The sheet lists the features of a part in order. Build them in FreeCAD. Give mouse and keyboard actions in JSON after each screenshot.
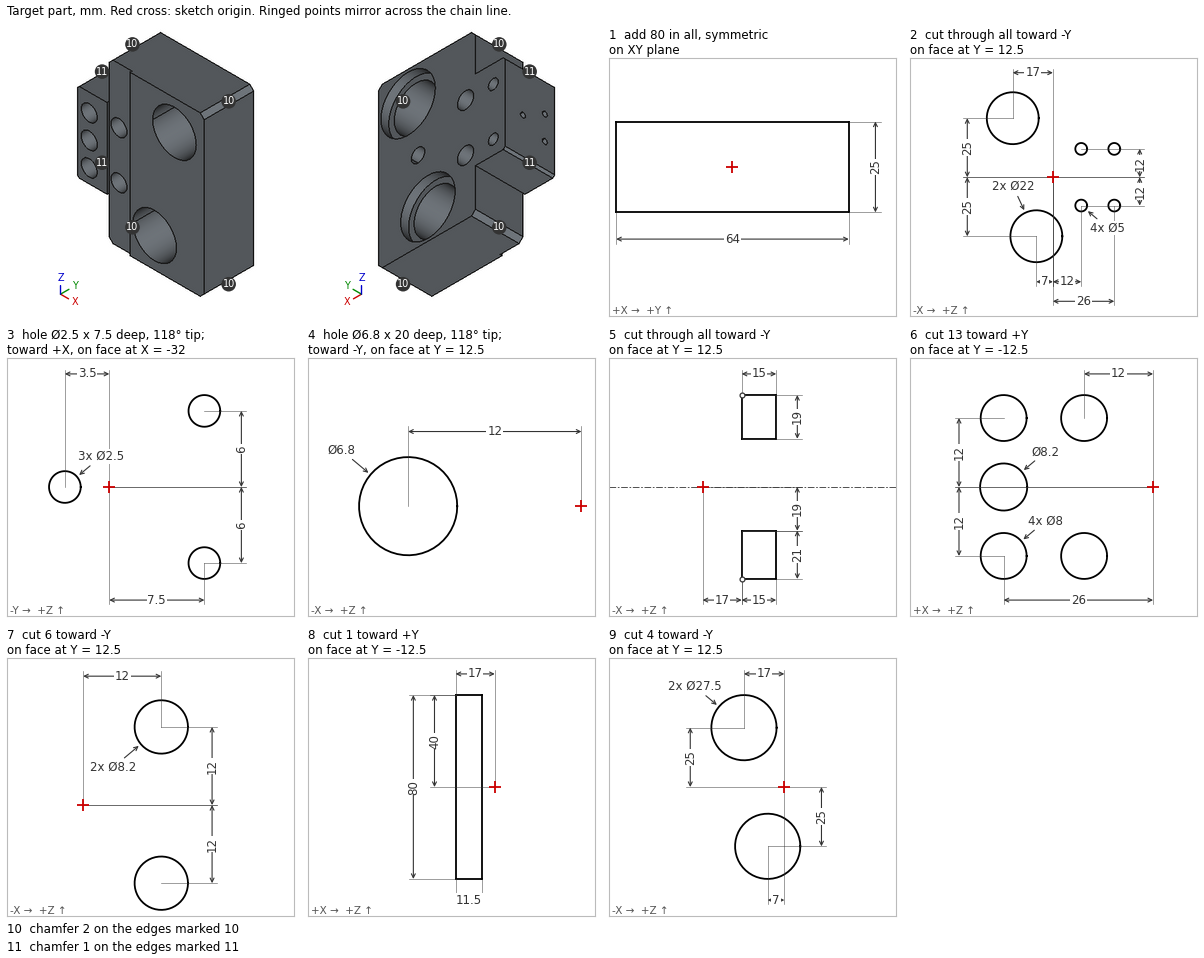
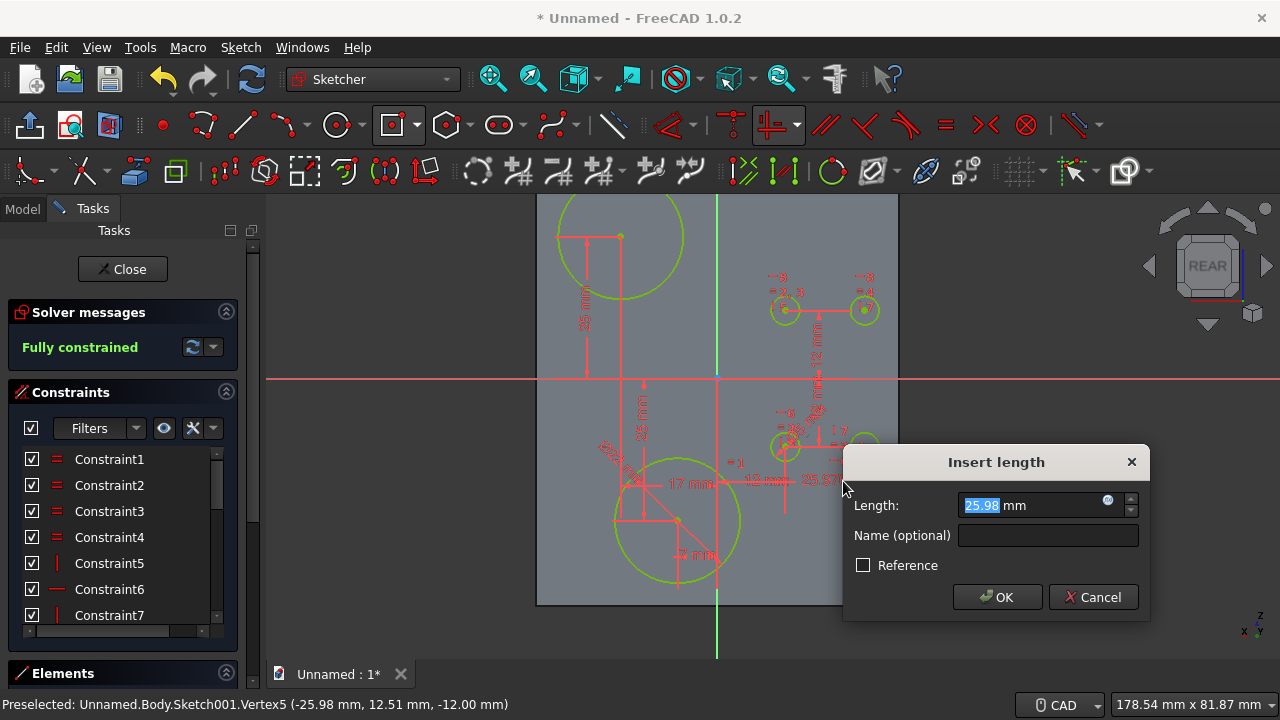
{"action": "type", "text": "26"}
{"action": "key", "text": "Return"}
{"action": "key", "text": "Escape"}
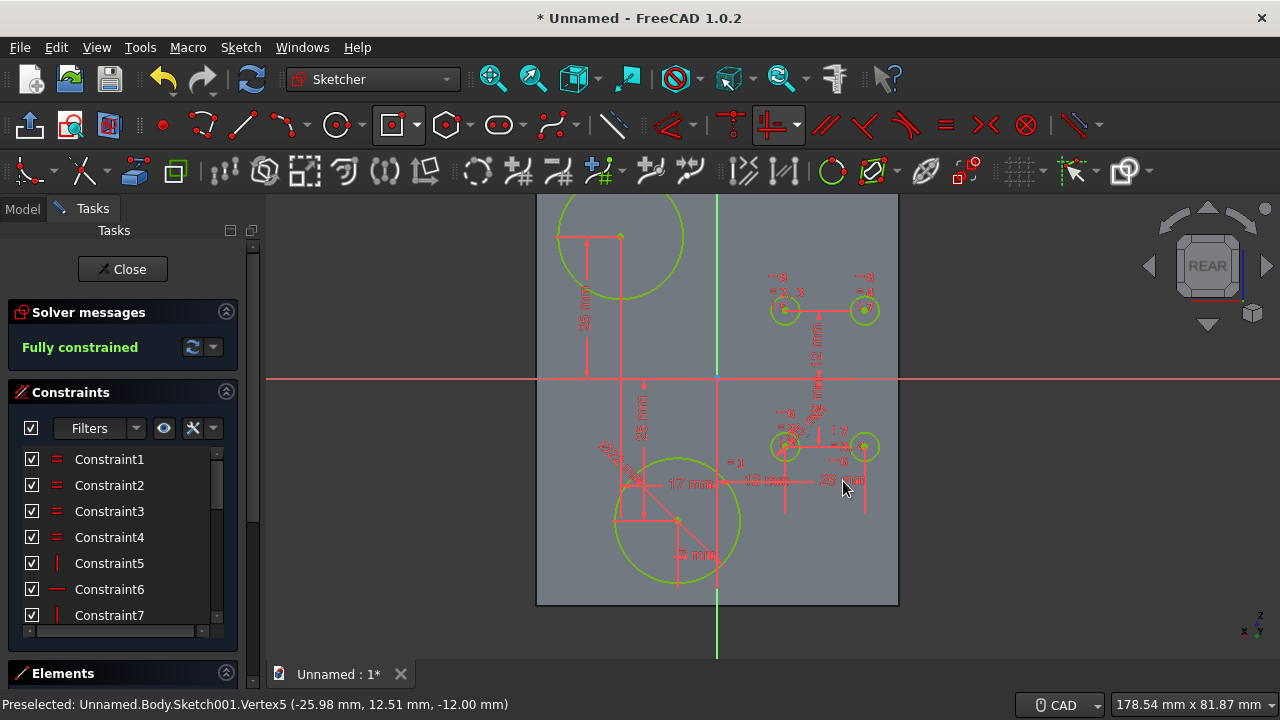
{"action": "left_click", "coordinate": [123, 269]}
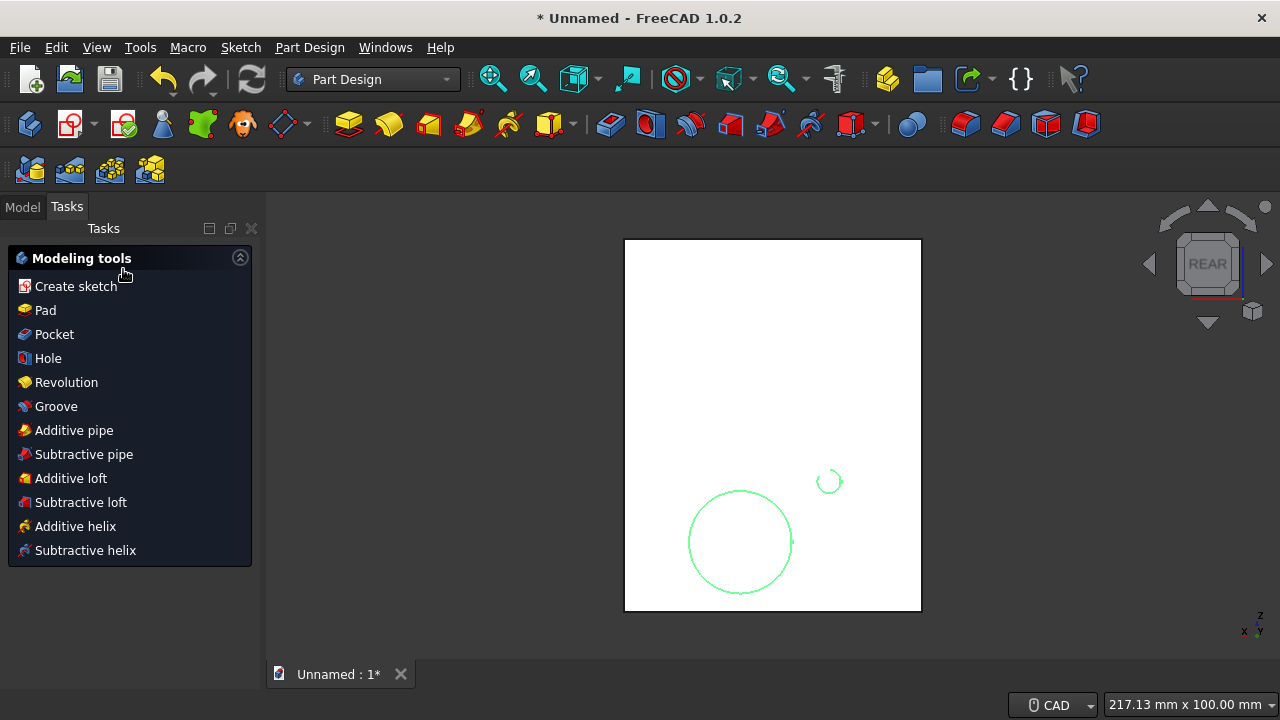
{"action": "left_click", "coordinate": [612, 124]}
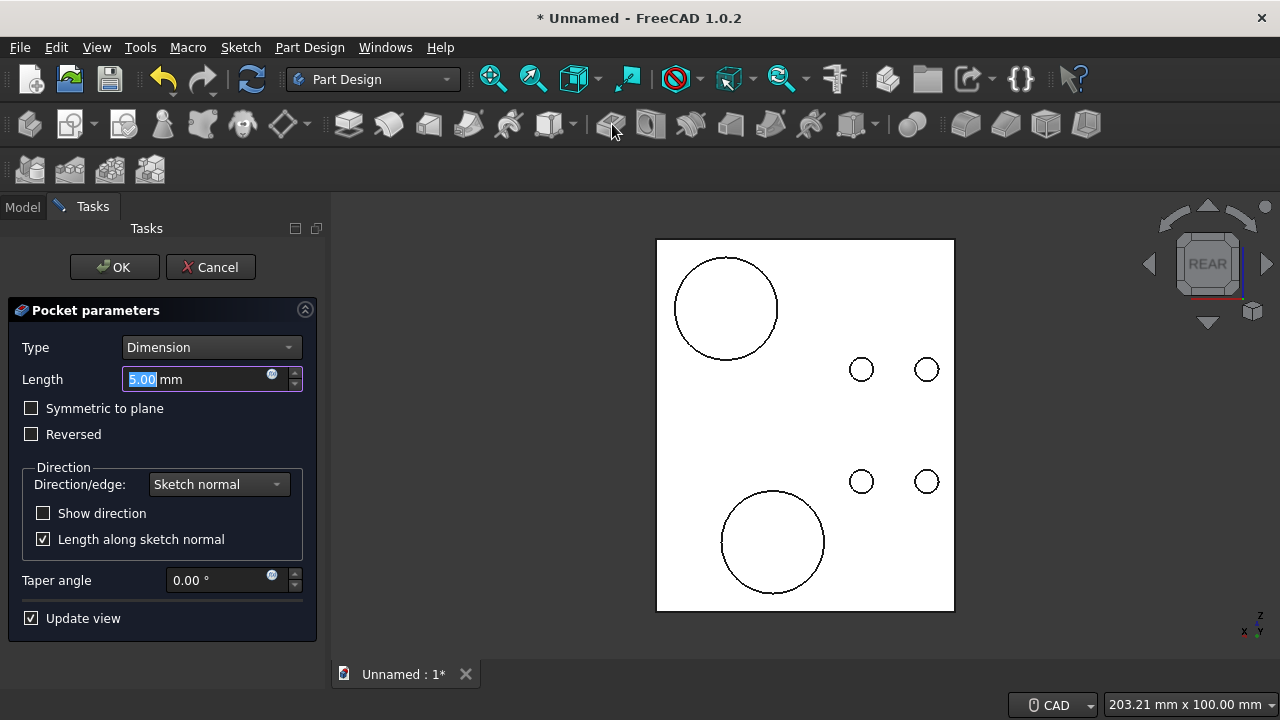
{"action": "left_click", "coordinate": [212, 348]}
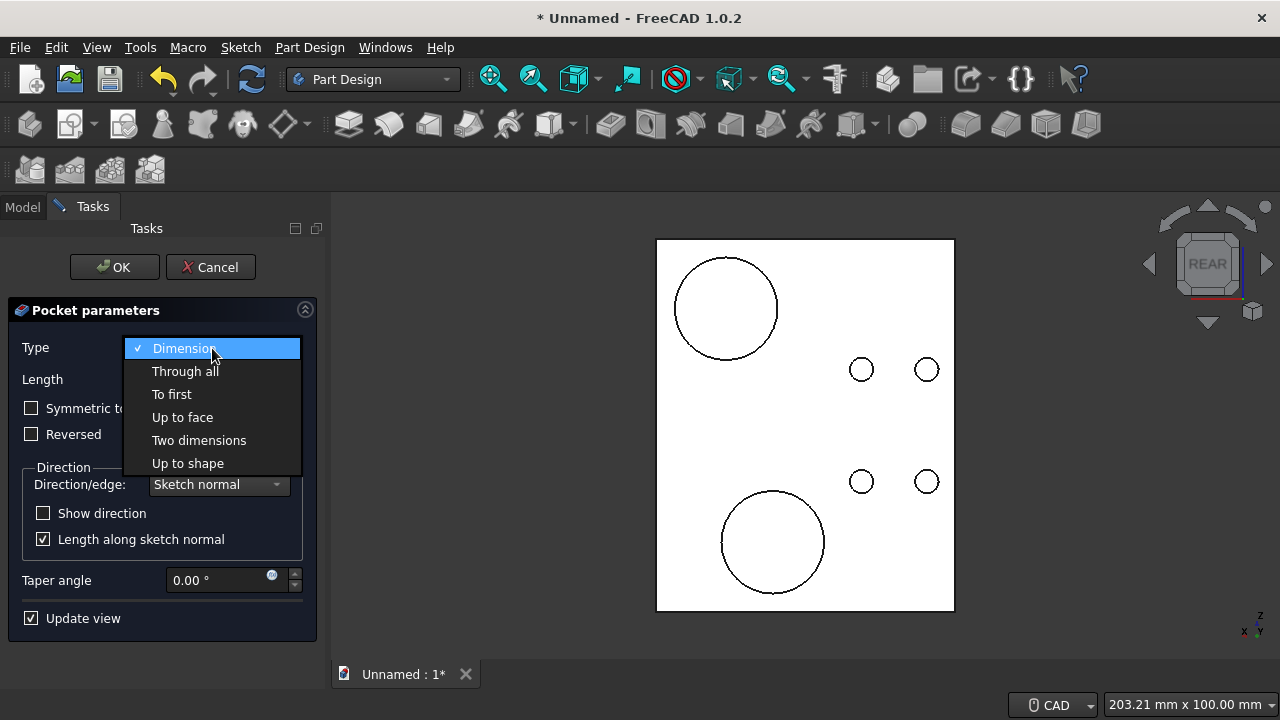
{"action": "left_click", "coordinate": [212, 372]}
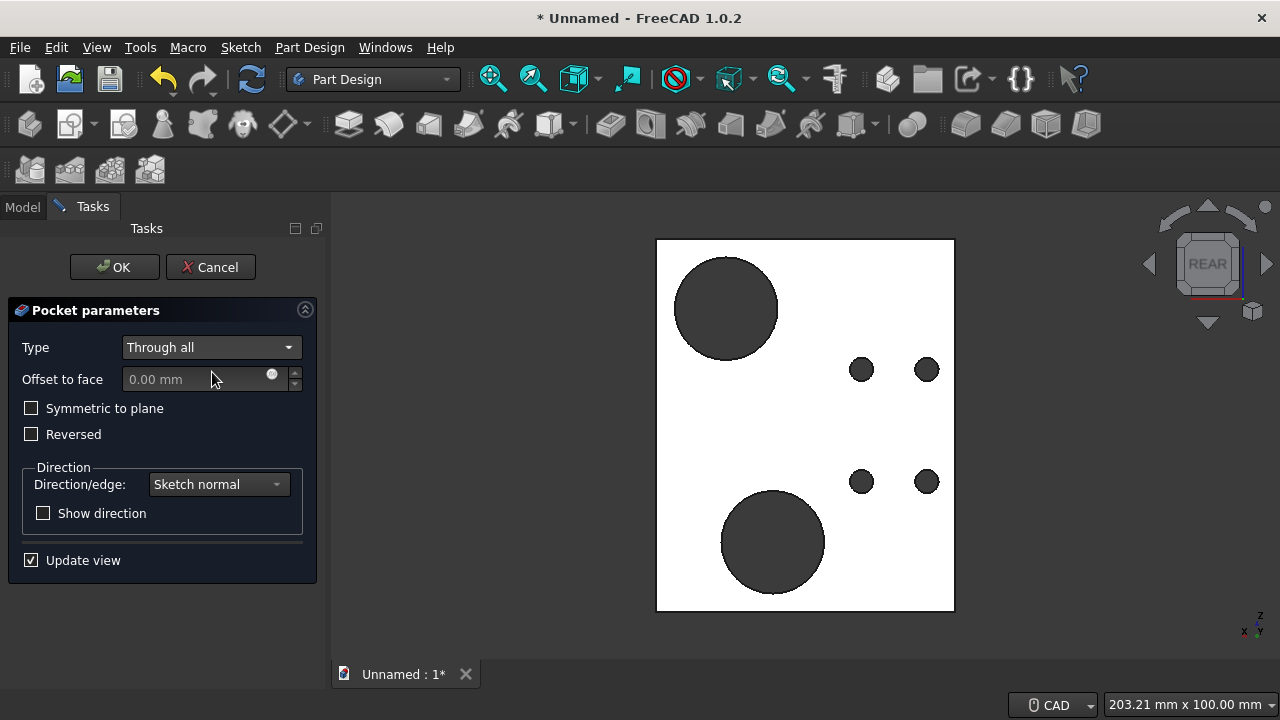
{"action": "left_click", "coordinate": [115, 267]}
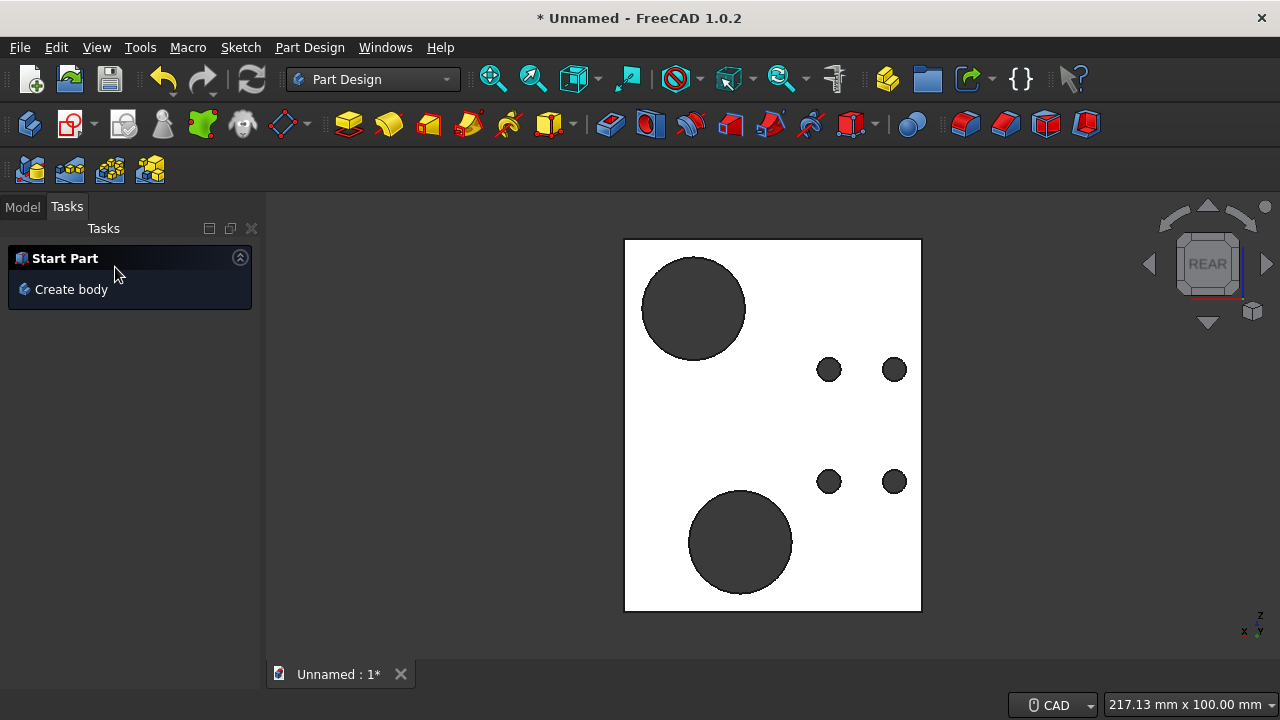
{"action": "key", "text": "6"}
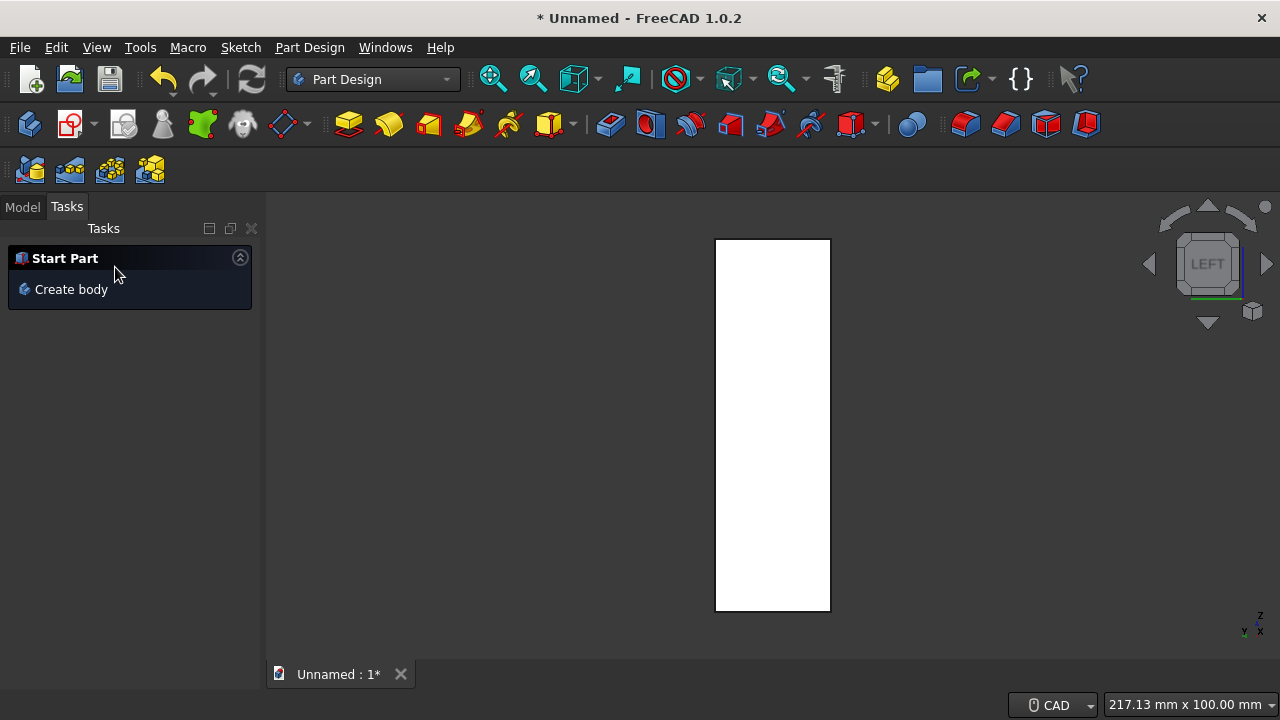
{"action": "left_click", "coordinate": [773, 318]}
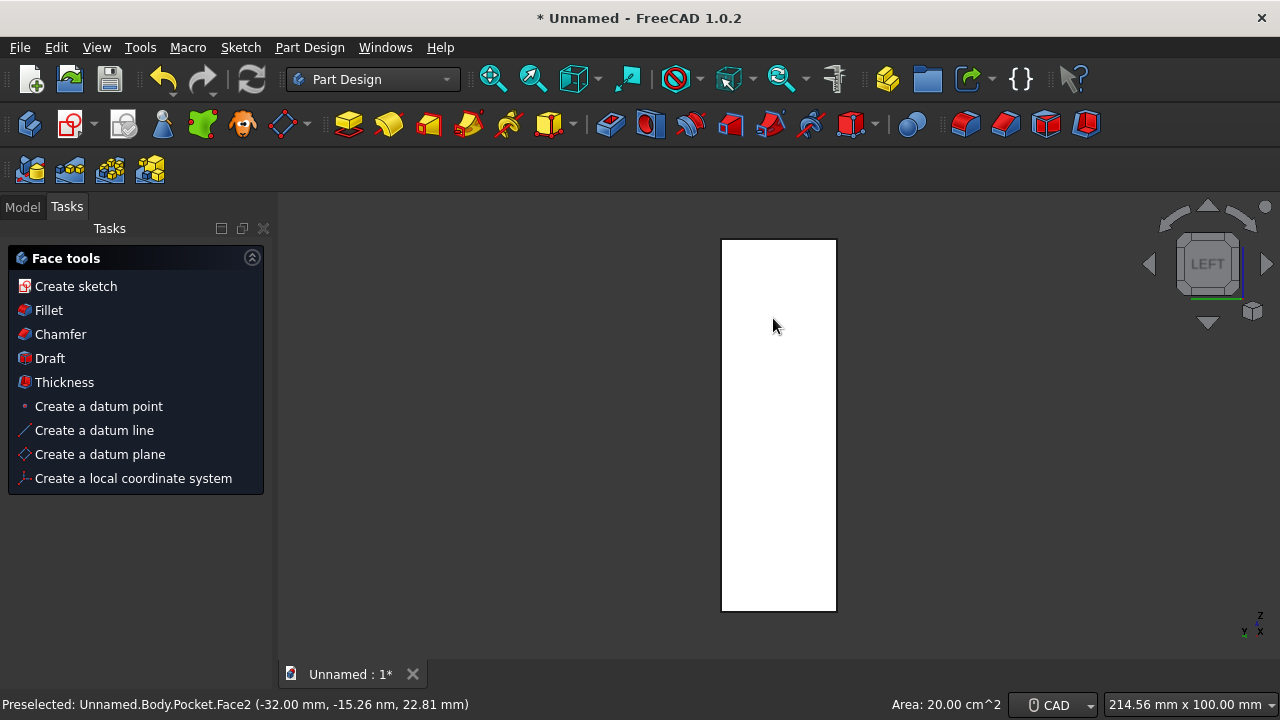
{"action": "left_click", "coordinate": [70, 124]}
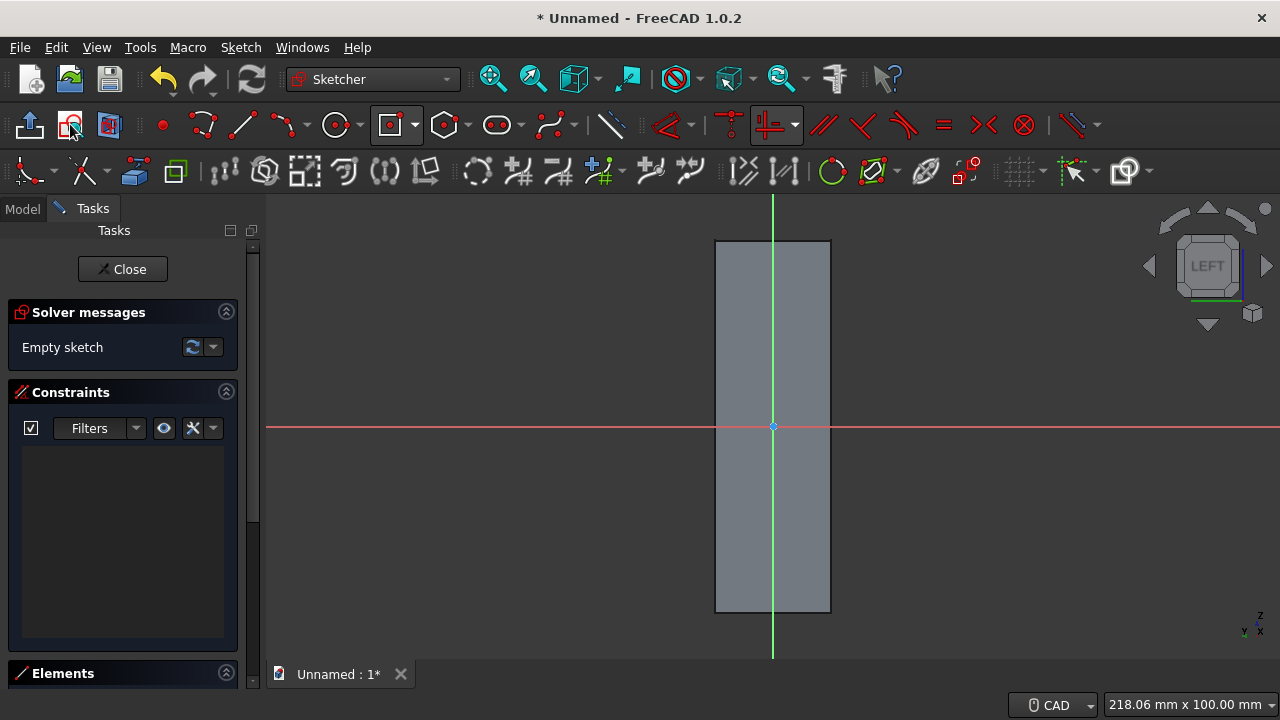
{"action": "scroll", "coordinate": [808, 427], "scroll_direction": "up", "scroll_amount": 7}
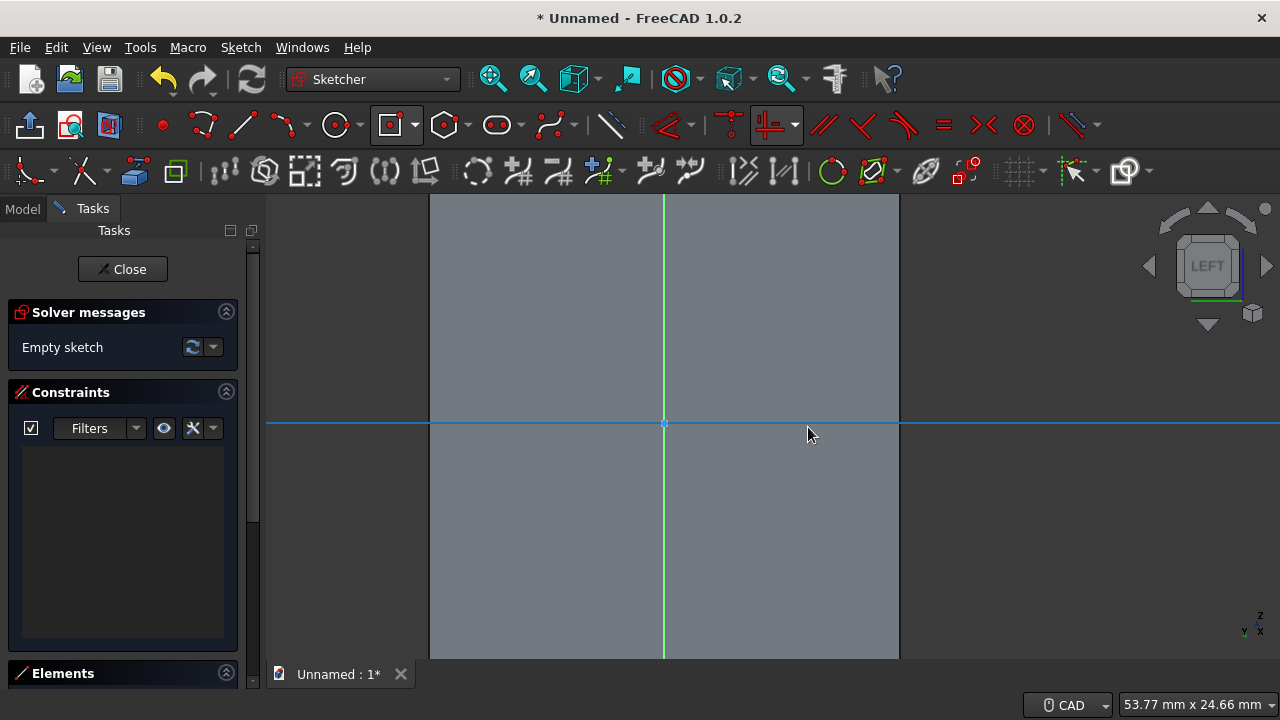
{"action": "left_click", "coordinate": [336, 126]}